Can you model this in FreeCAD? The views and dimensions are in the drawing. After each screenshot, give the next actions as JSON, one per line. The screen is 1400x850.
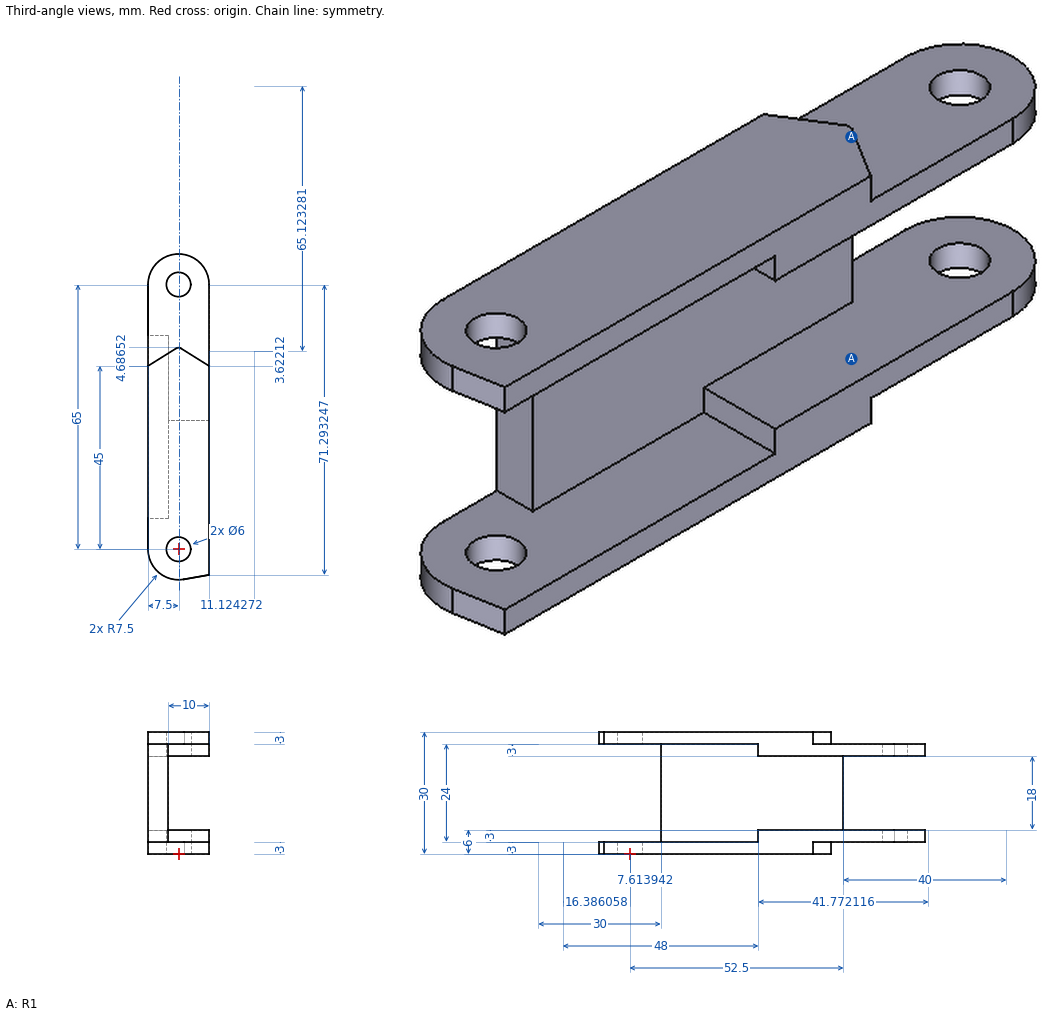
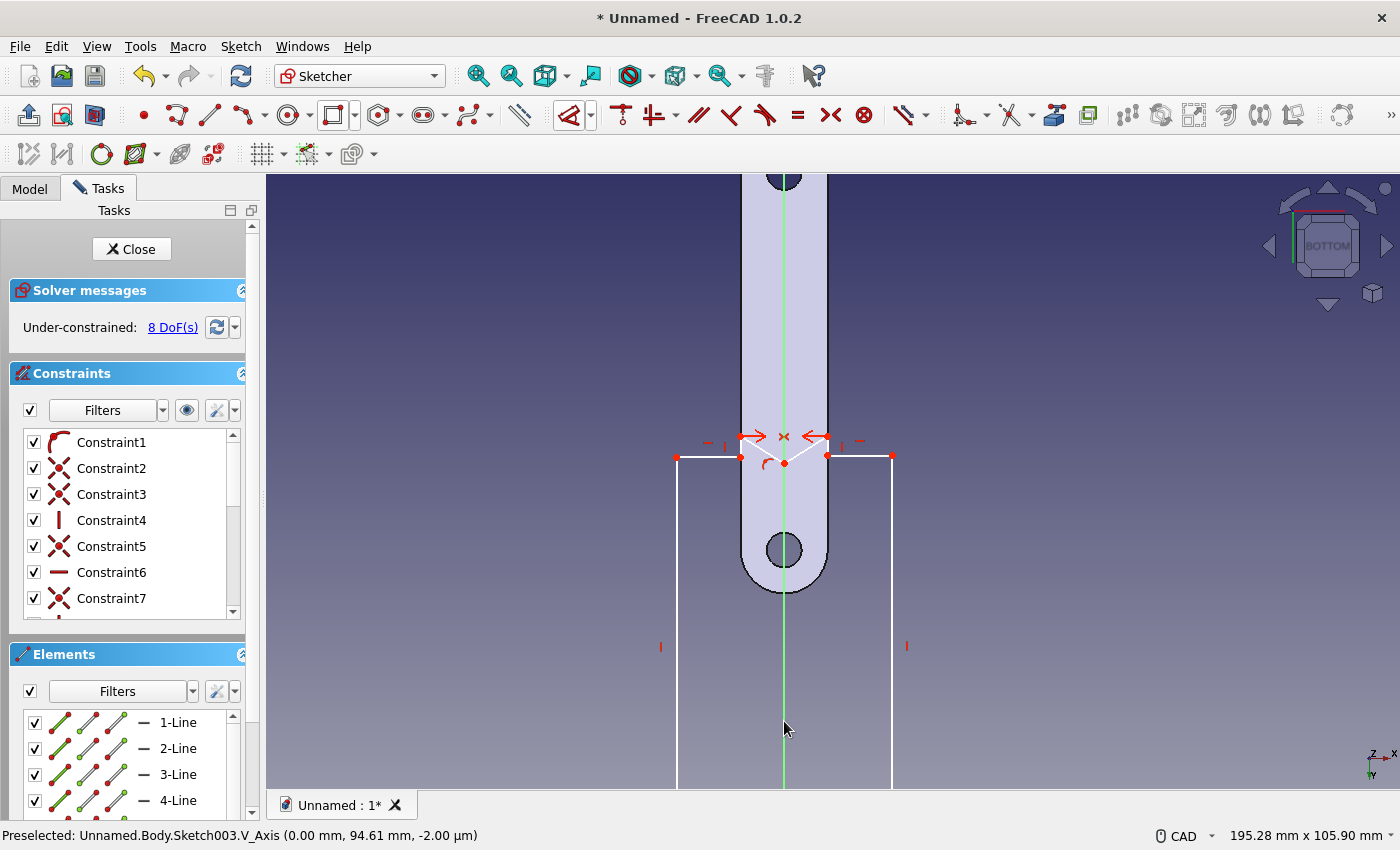
{"action": "left_click", "coordinate": [892, 456]}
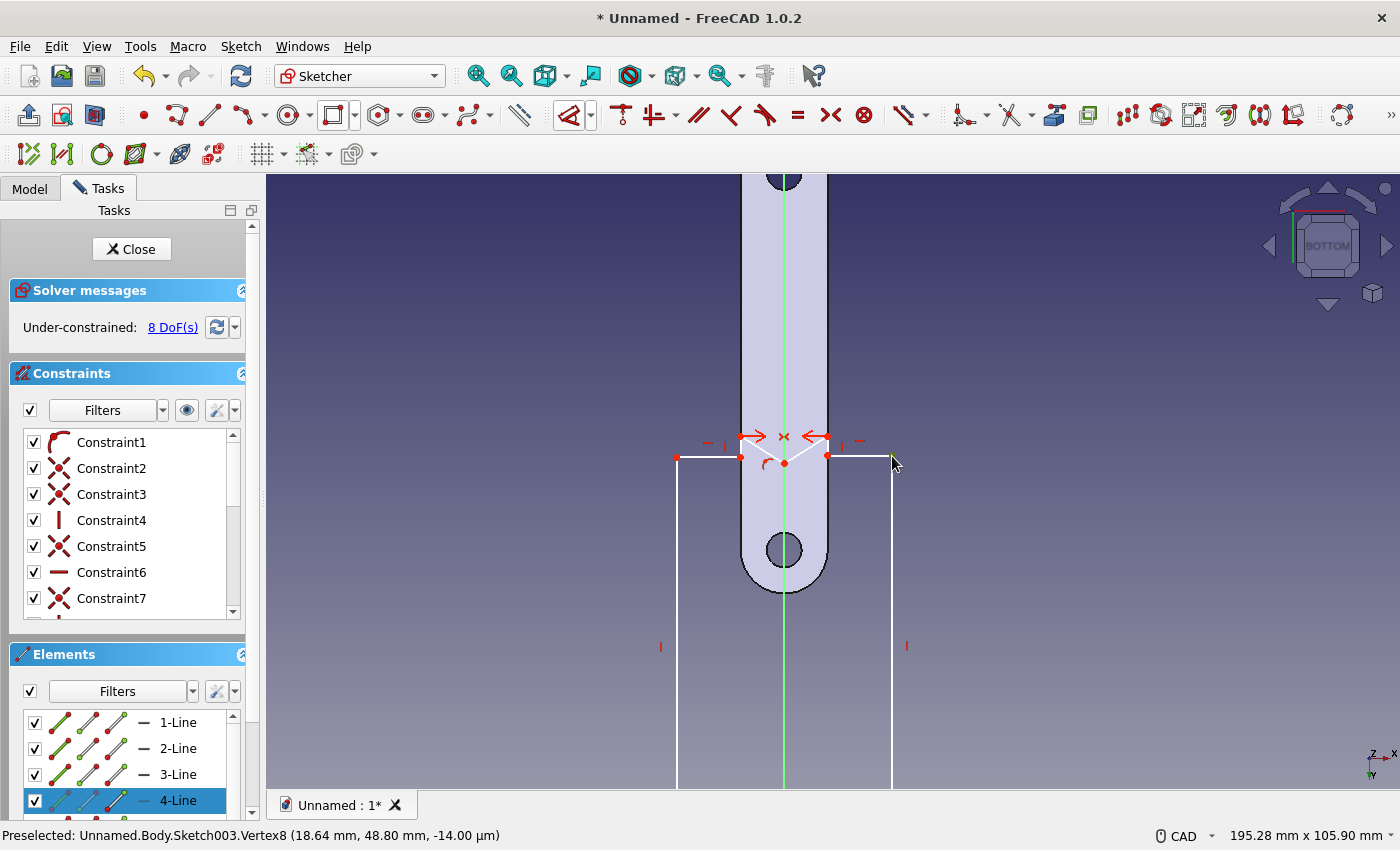
{"action": "left_click", "coordinate": [677, 457]}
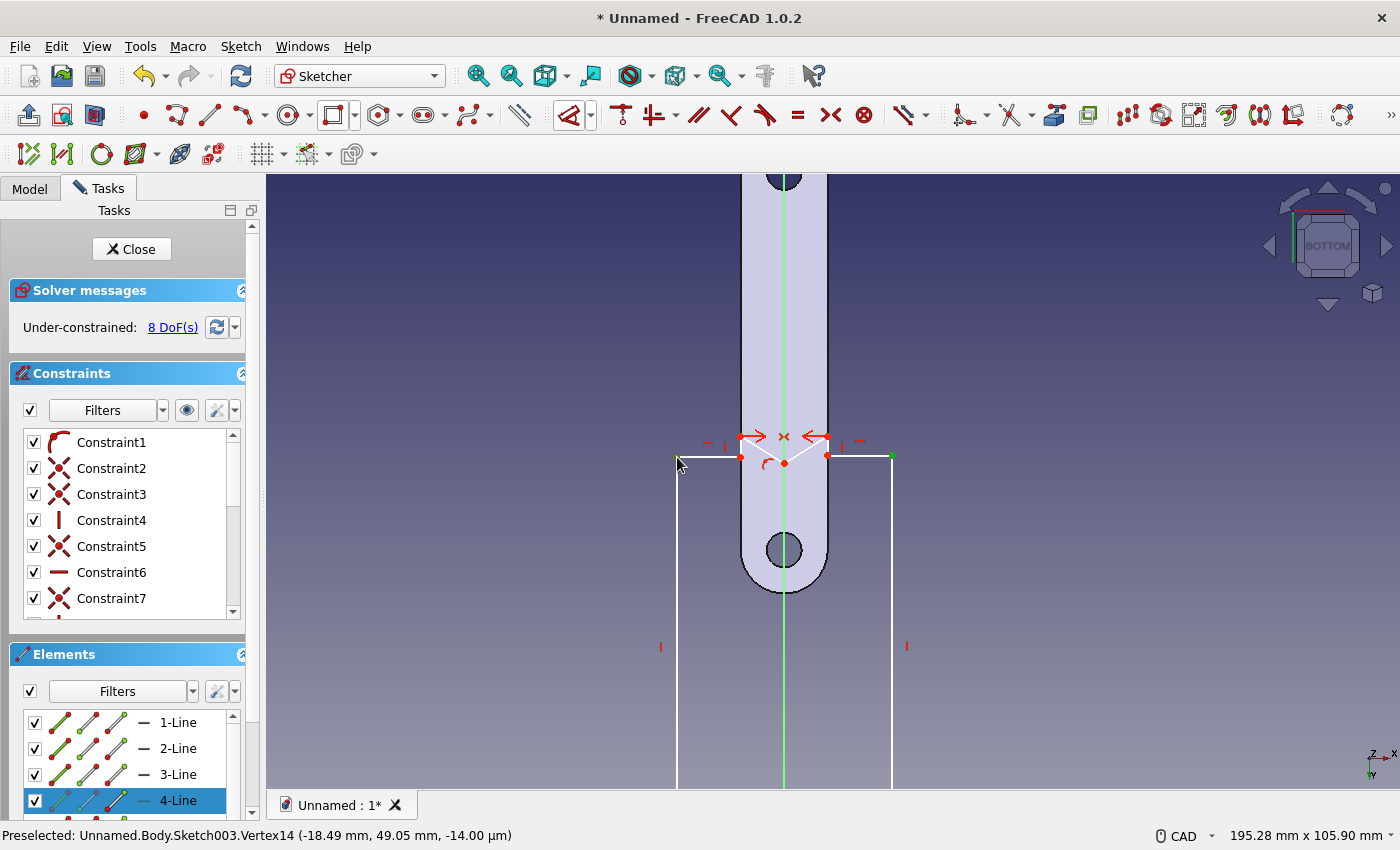
{"action": "left_click", "coordinate": [784, 721]}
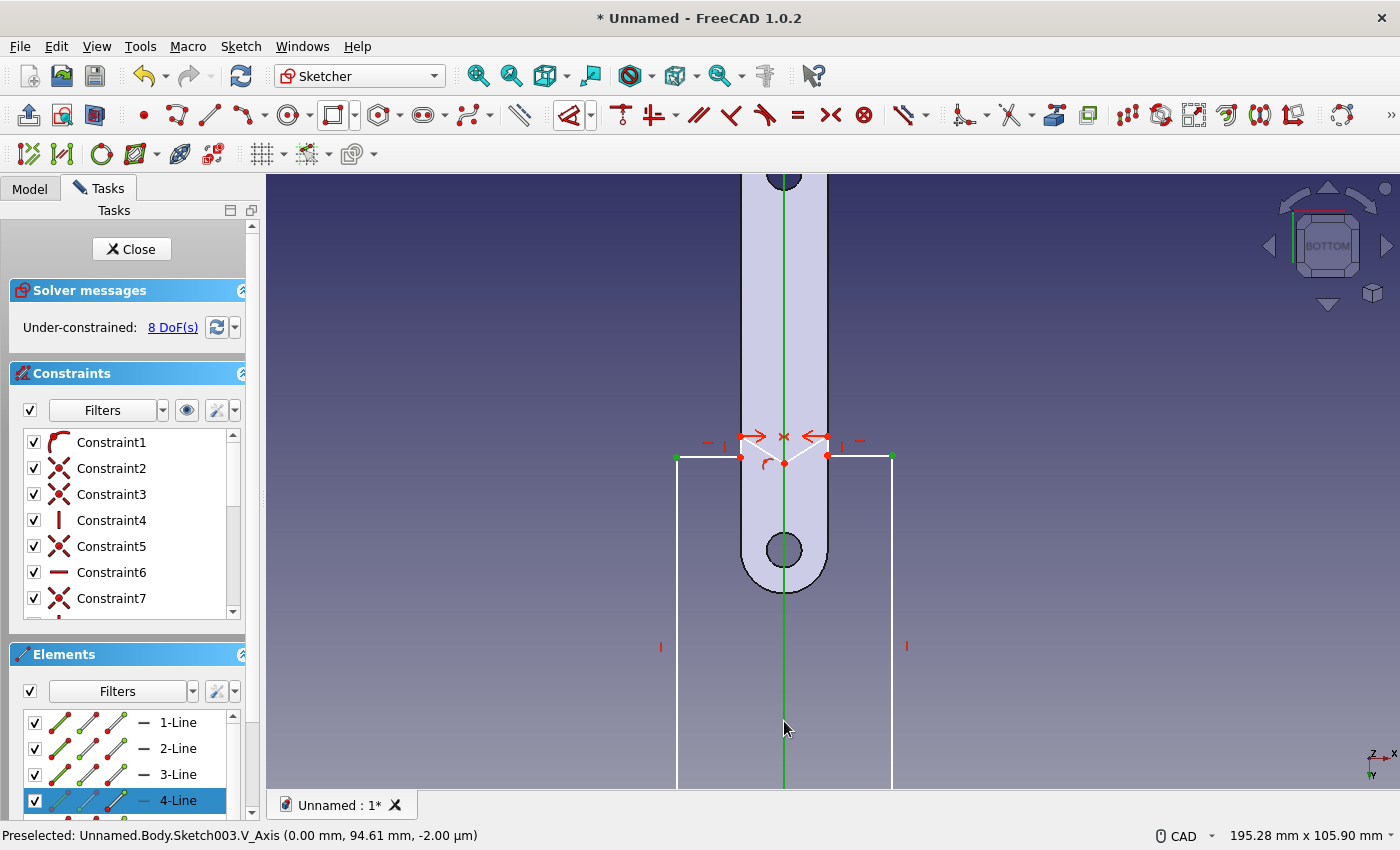
{"action": "key", "text": "s"}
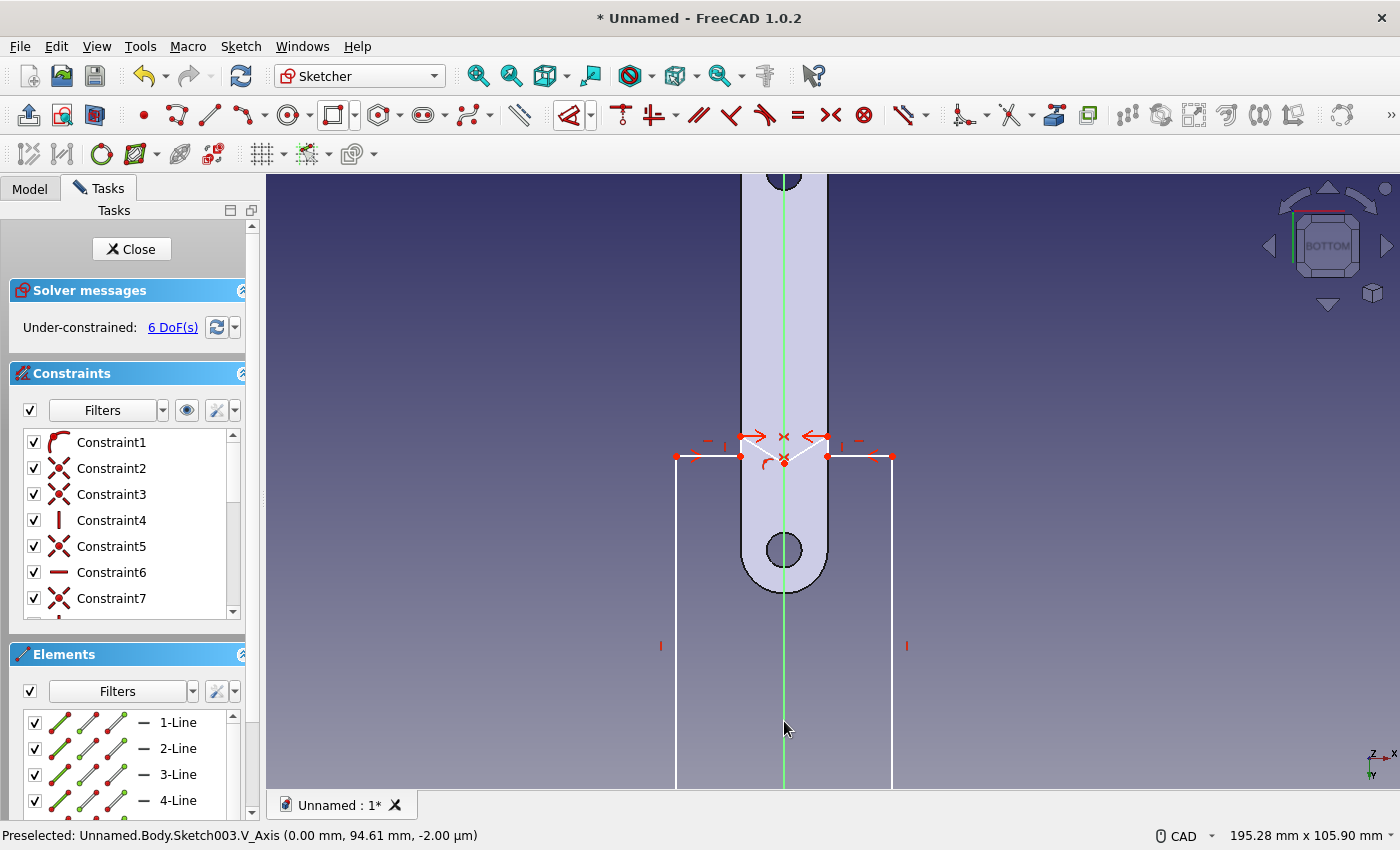
{"action": "left_click", "coordinate": [741, 436]}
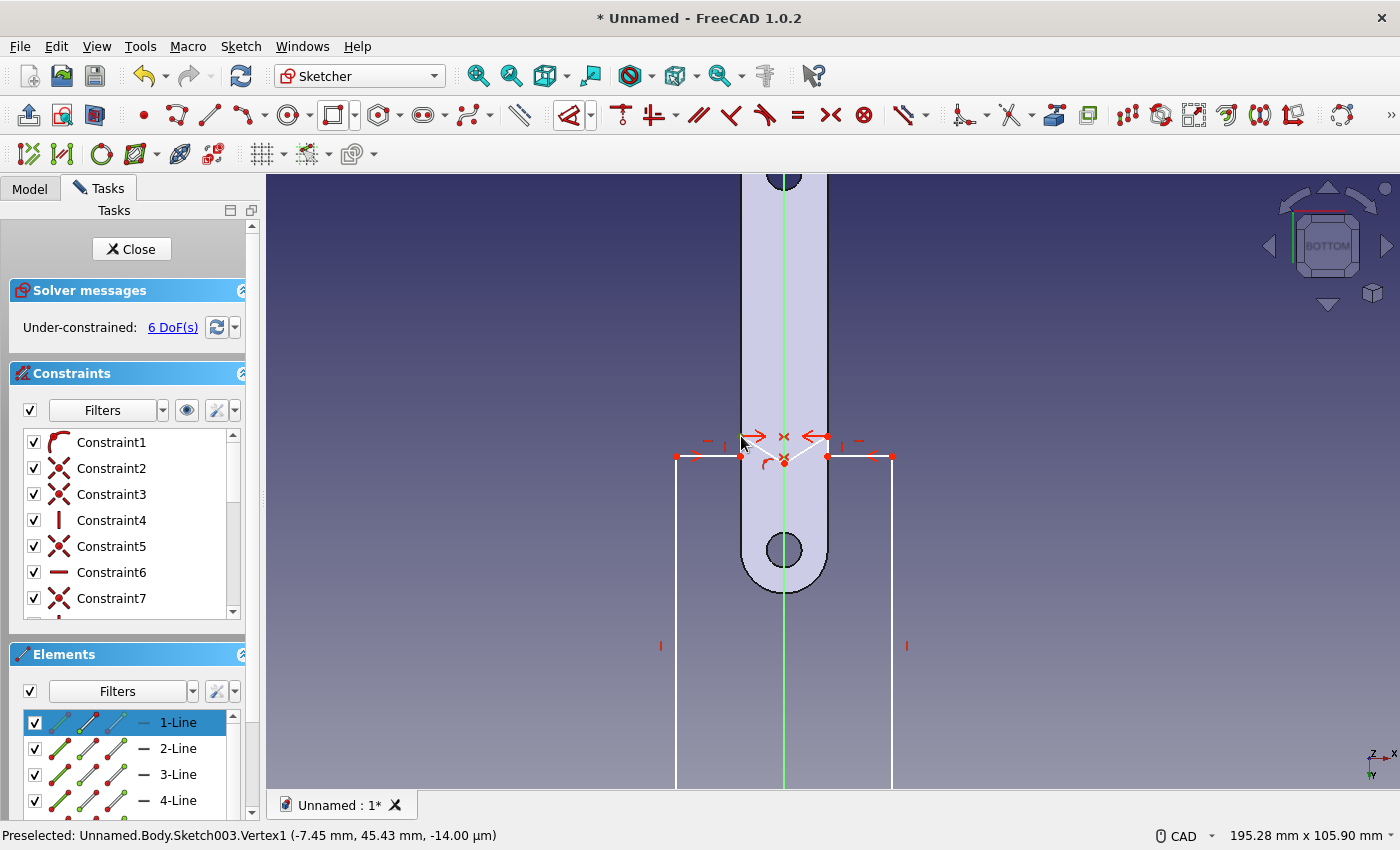
{"action": "left_click", "coordinate": [590, 116]}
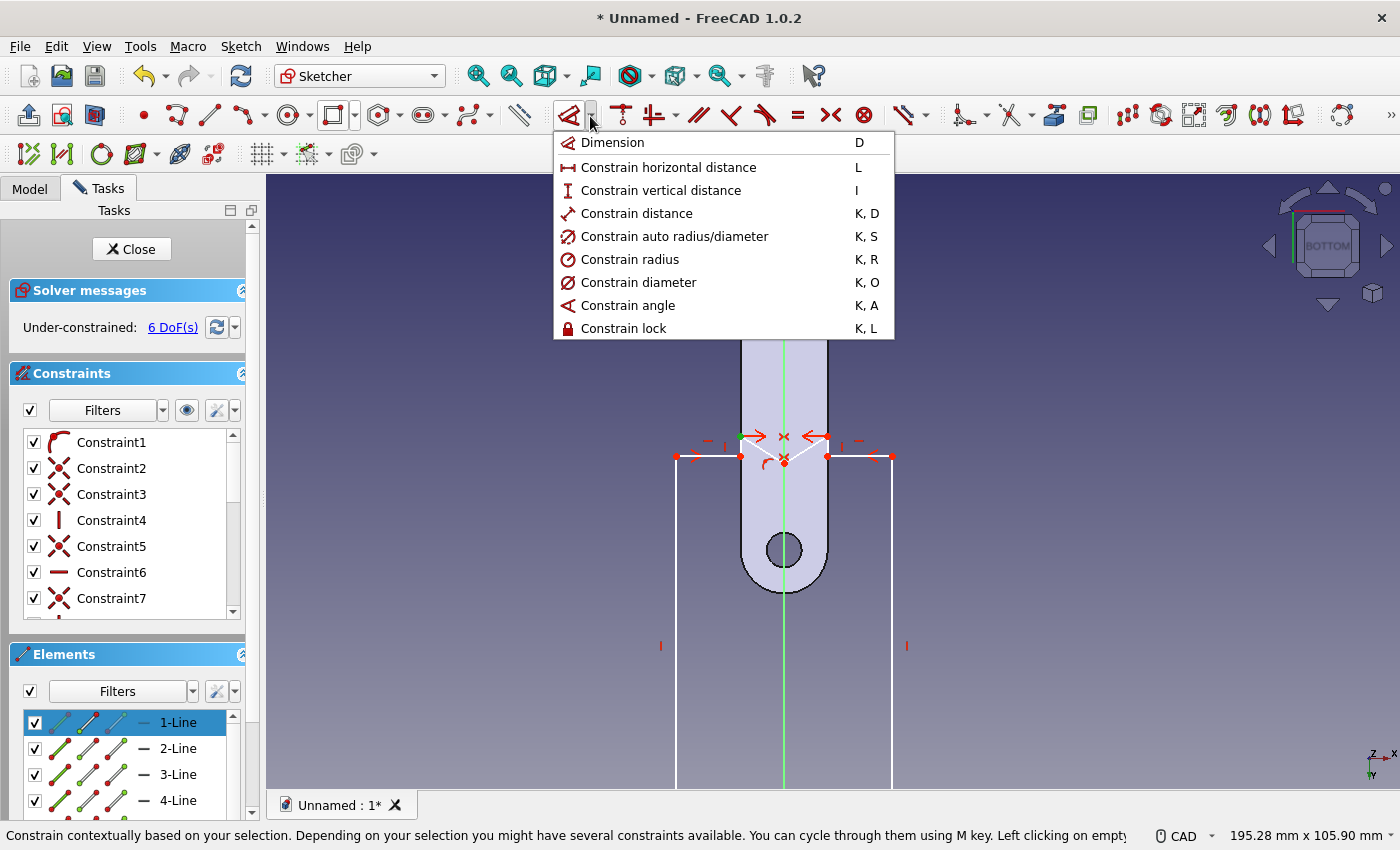
{"action": "left_click", "coordinate": [724, 190]}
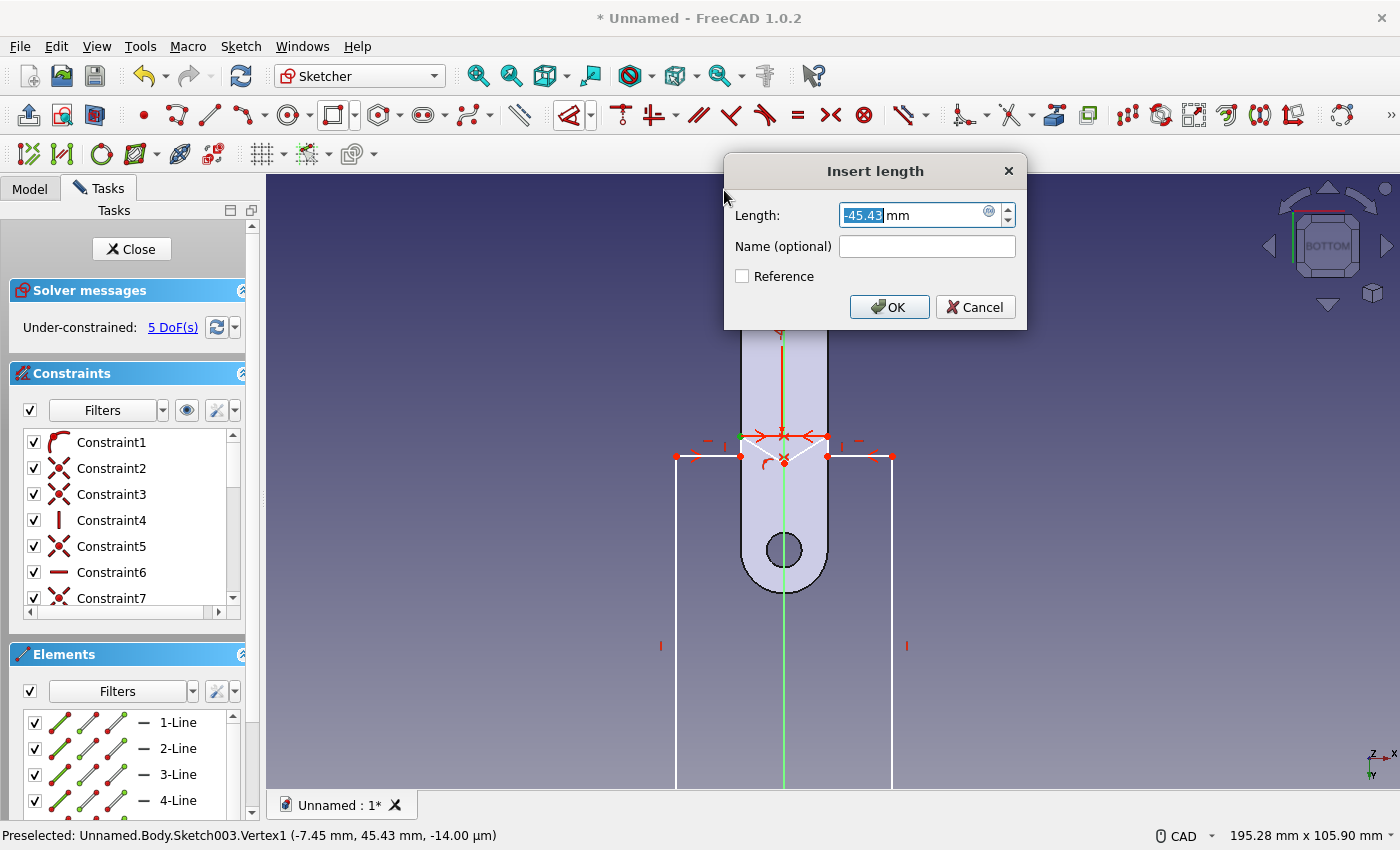
{"action": "type", "text": "-45"}
{"action": "key", "text": "Return"}